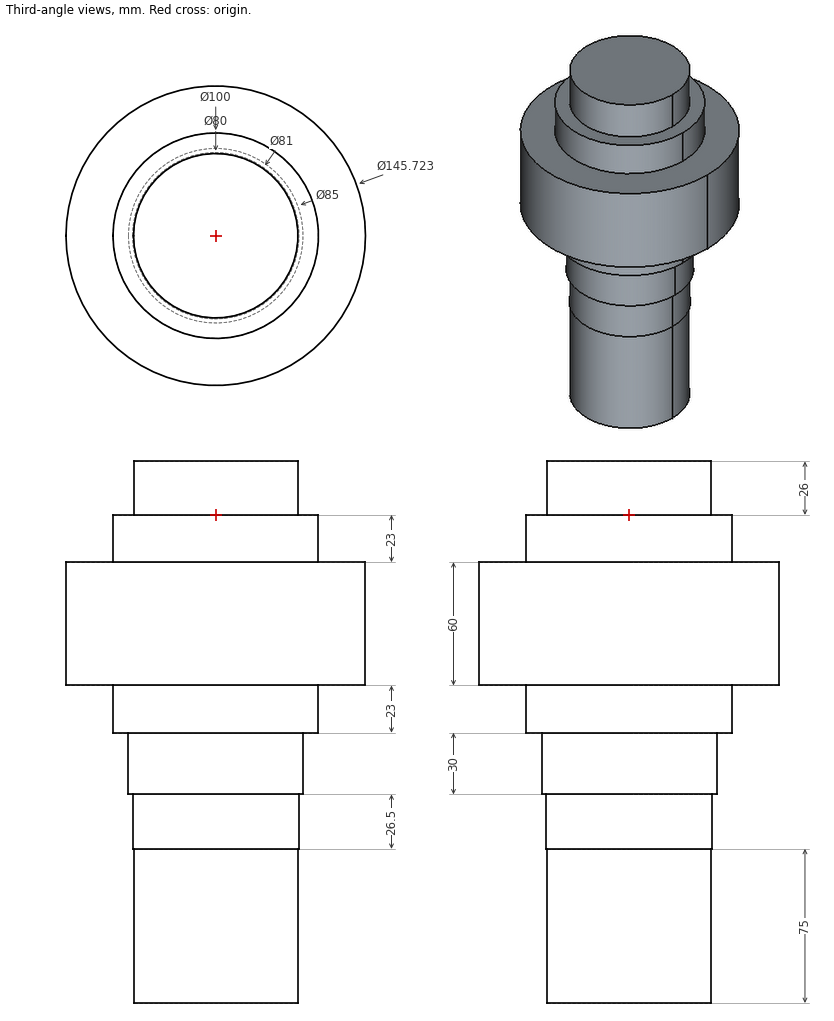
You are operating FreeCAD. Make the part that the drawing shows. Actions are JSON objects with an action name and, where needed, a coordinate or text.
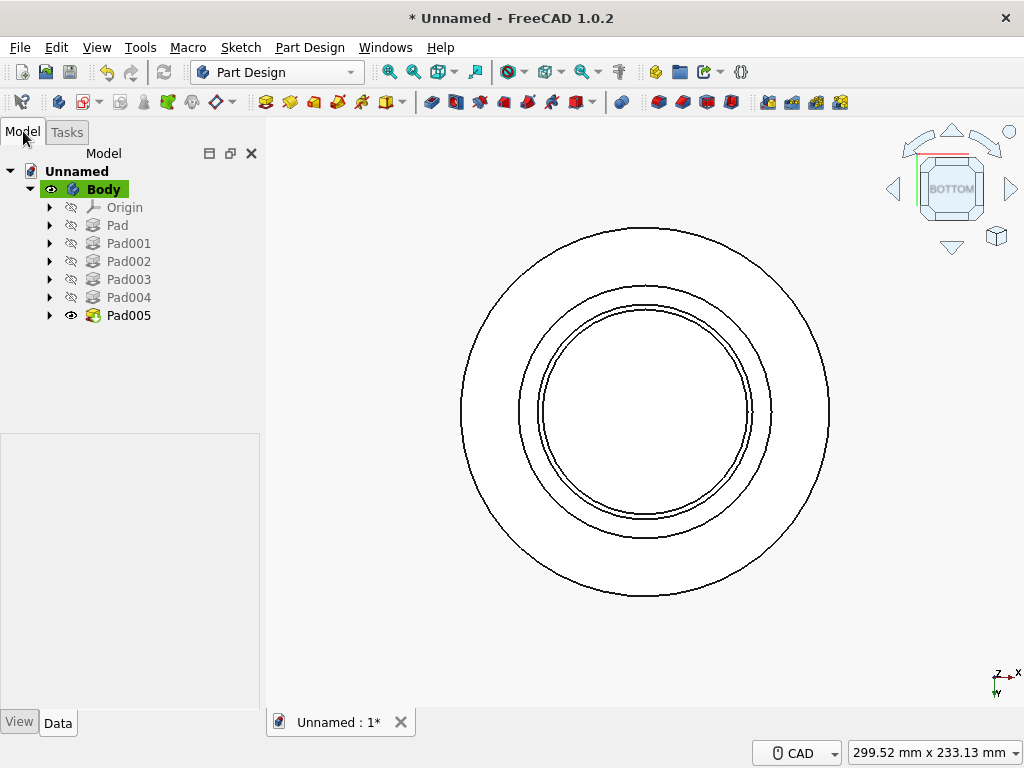
{"action": "left_click", "coordinate": [50, 207]}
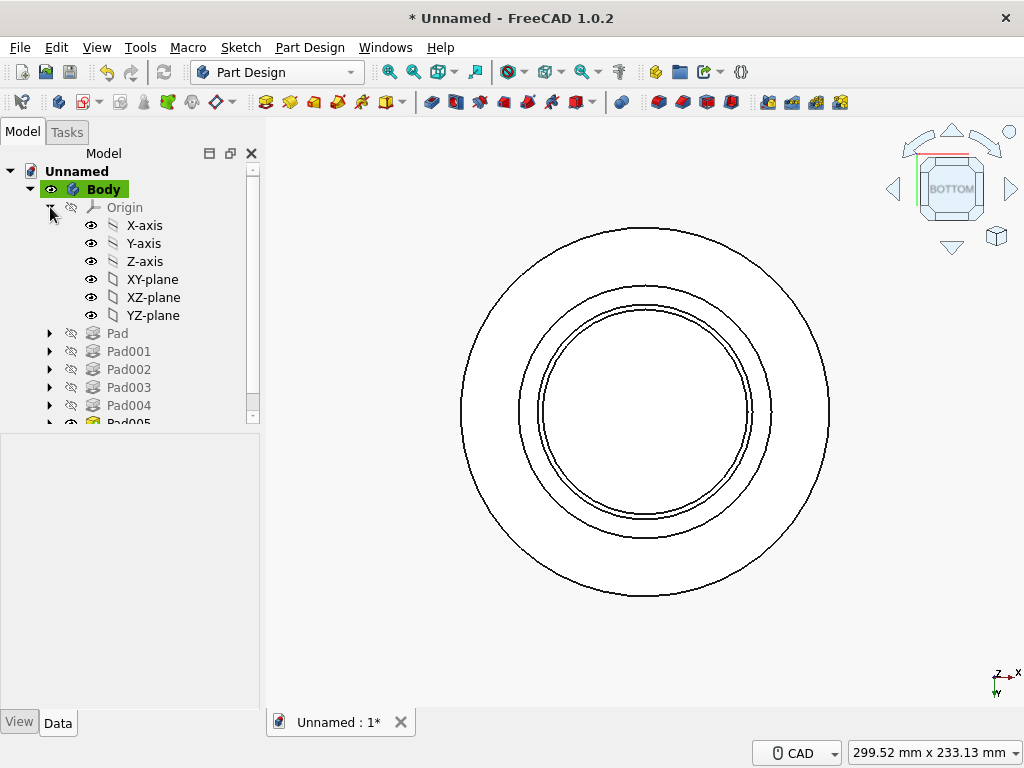
{"action": "left_click", "coordinate": [136, 279]}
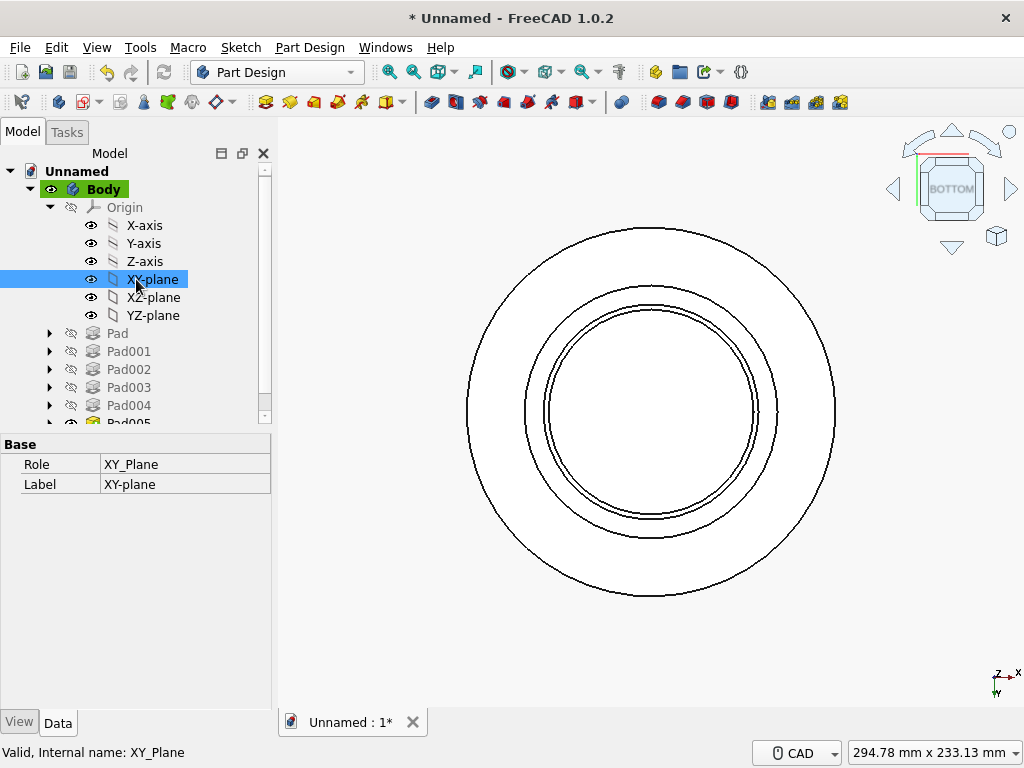
{"action": "left_click", "coordinate": [216, 102]}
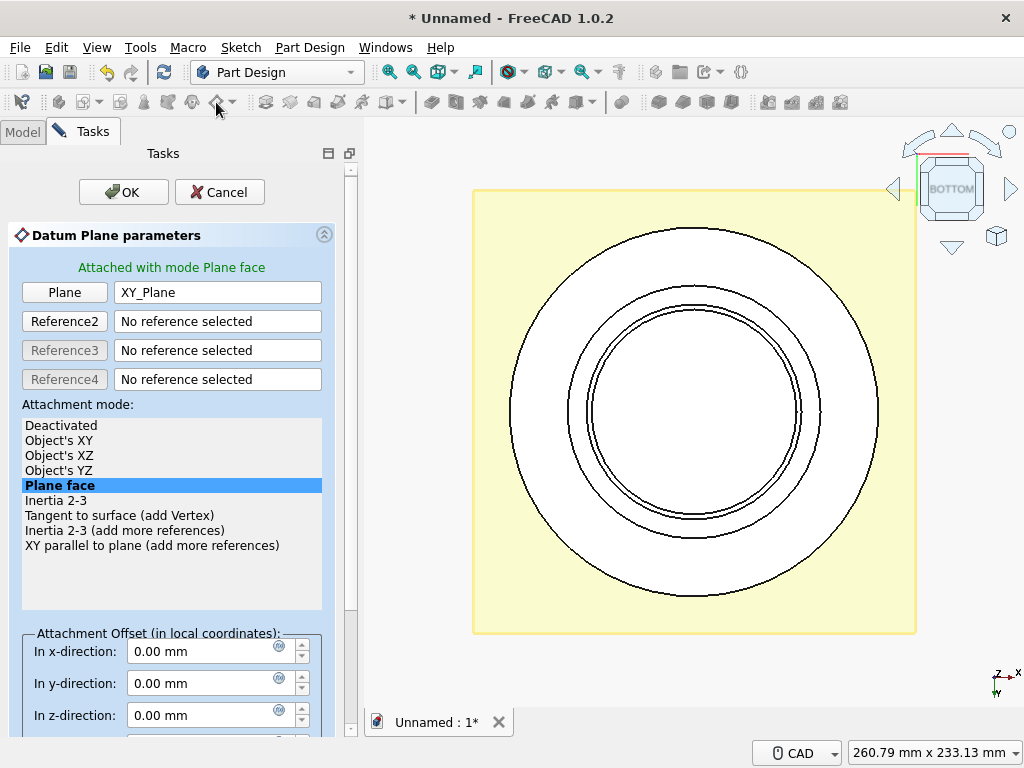
{"action": "triple_click", "coordinate": [210, 715]}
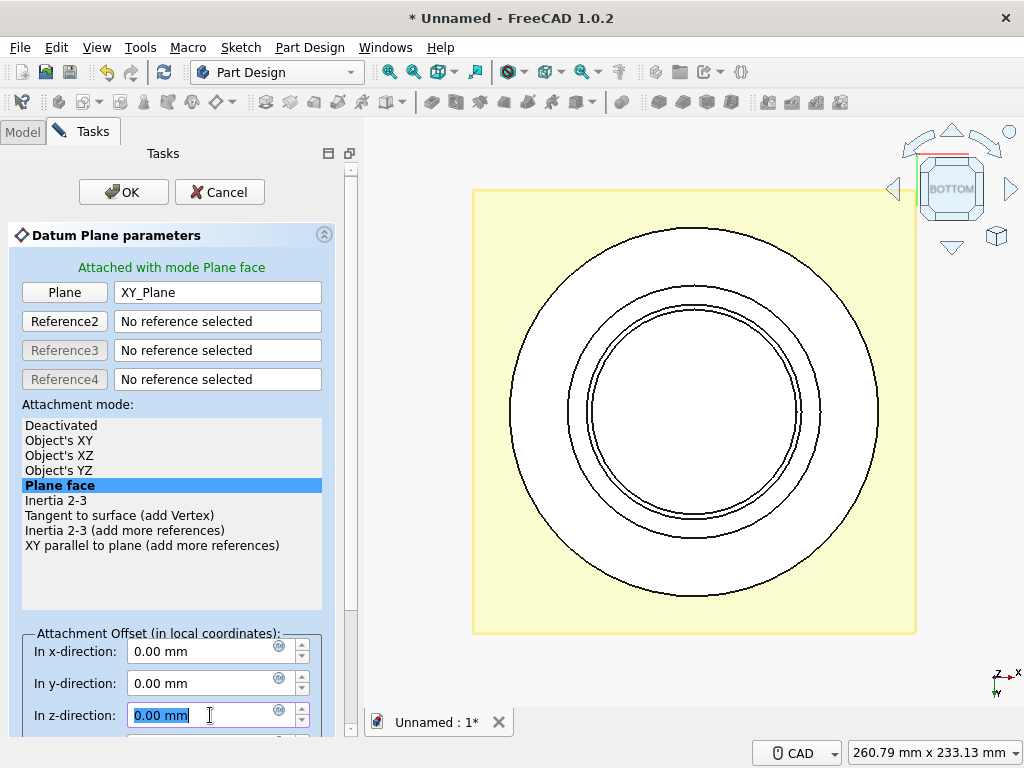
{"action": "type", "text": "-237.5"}
{"action": "key", "text": "Tab"}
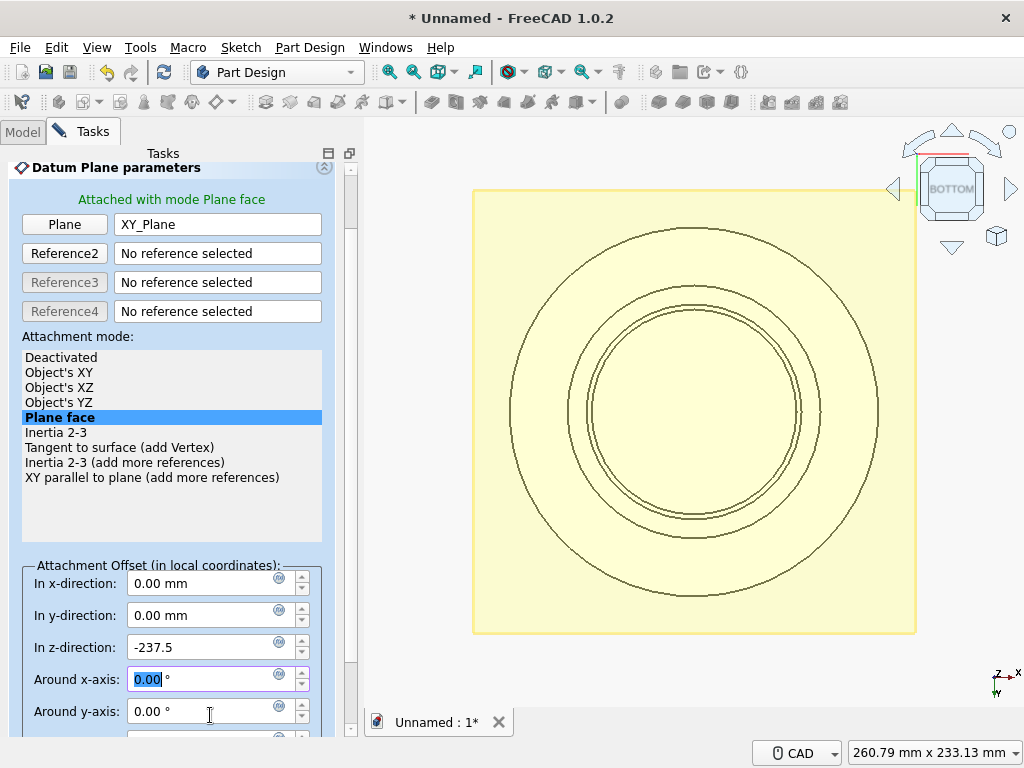
{"action": "scroll", "coordinate": [351, 450], "scroll_direction": "up", "scroll_amount": 2}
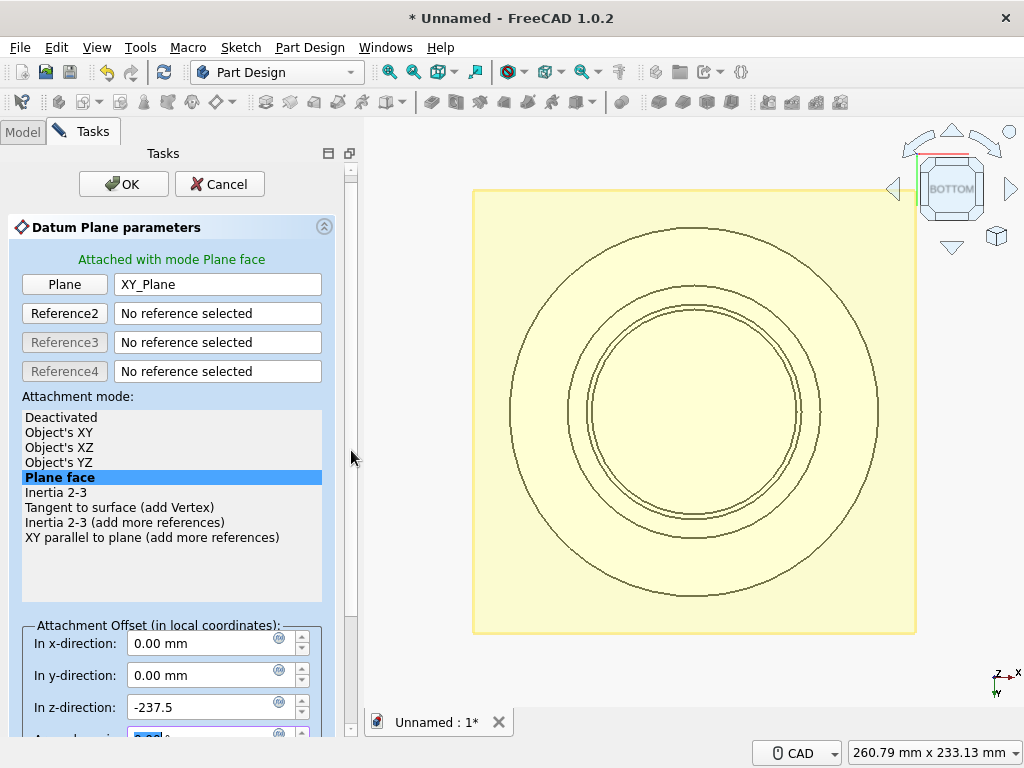
{"action": "left_click", "coordinate": [124, 192]}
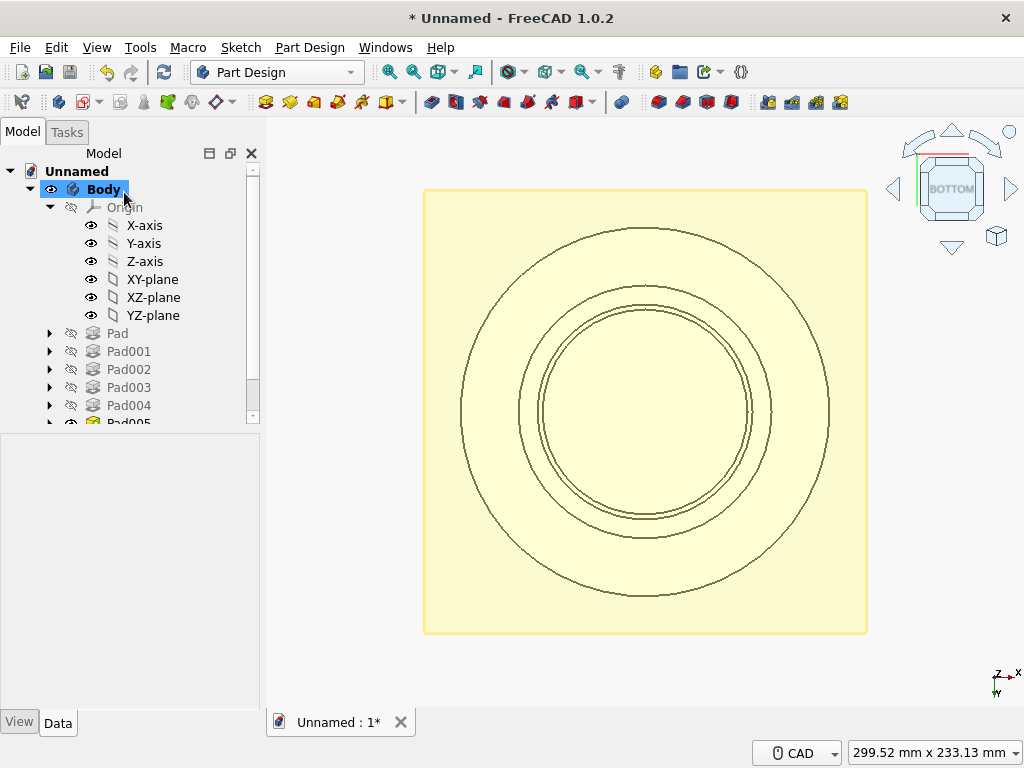
{"action": "scroll", "coordinate": [100, 293], "scroll_direction": "down", "scroll_amount": 3}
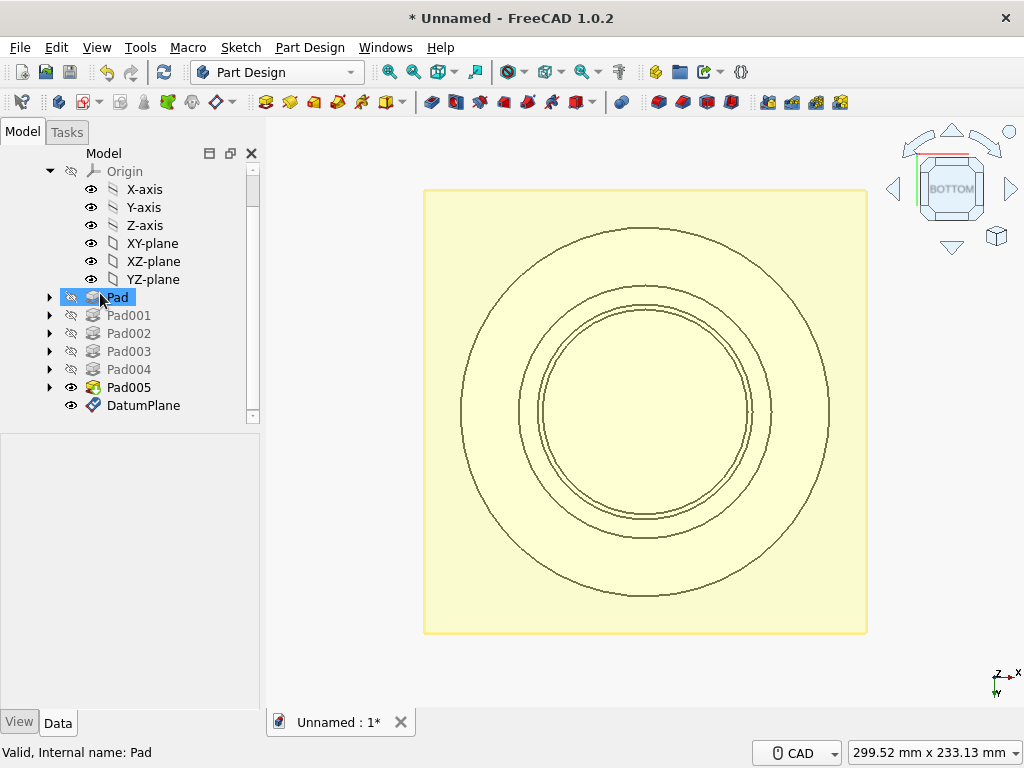
{"action": "left_click", "coordinate": [116, 405]}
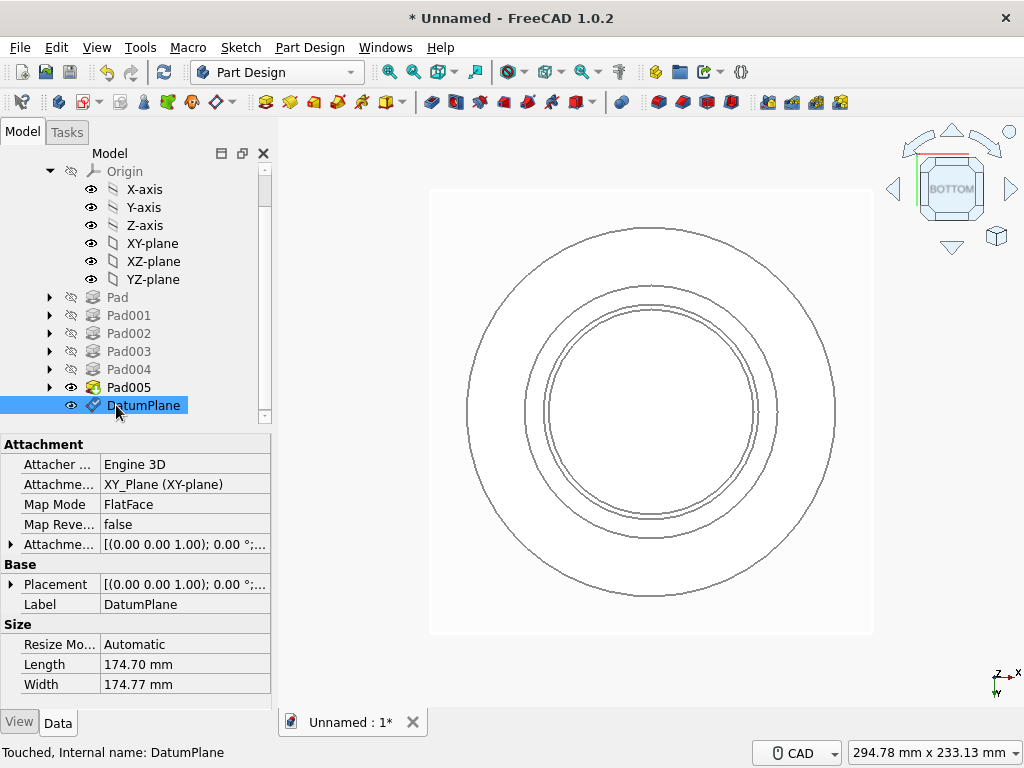
{"action": "left_click", "coordinate": [84, 102]}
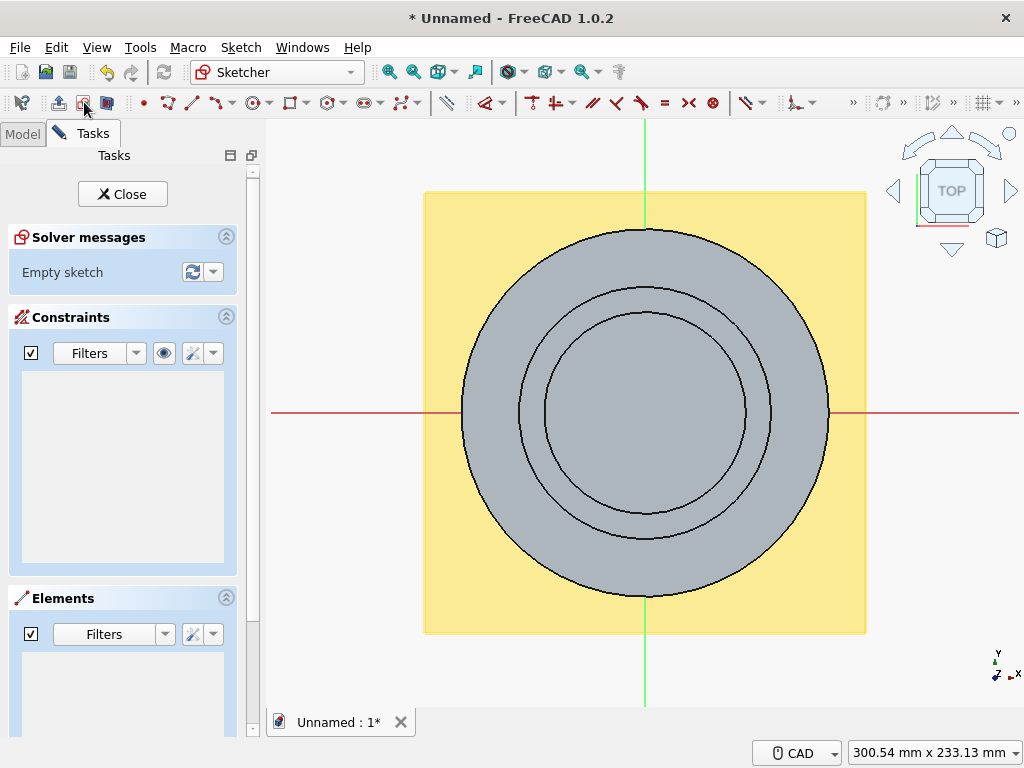
{"action": "key", "text": "q s"}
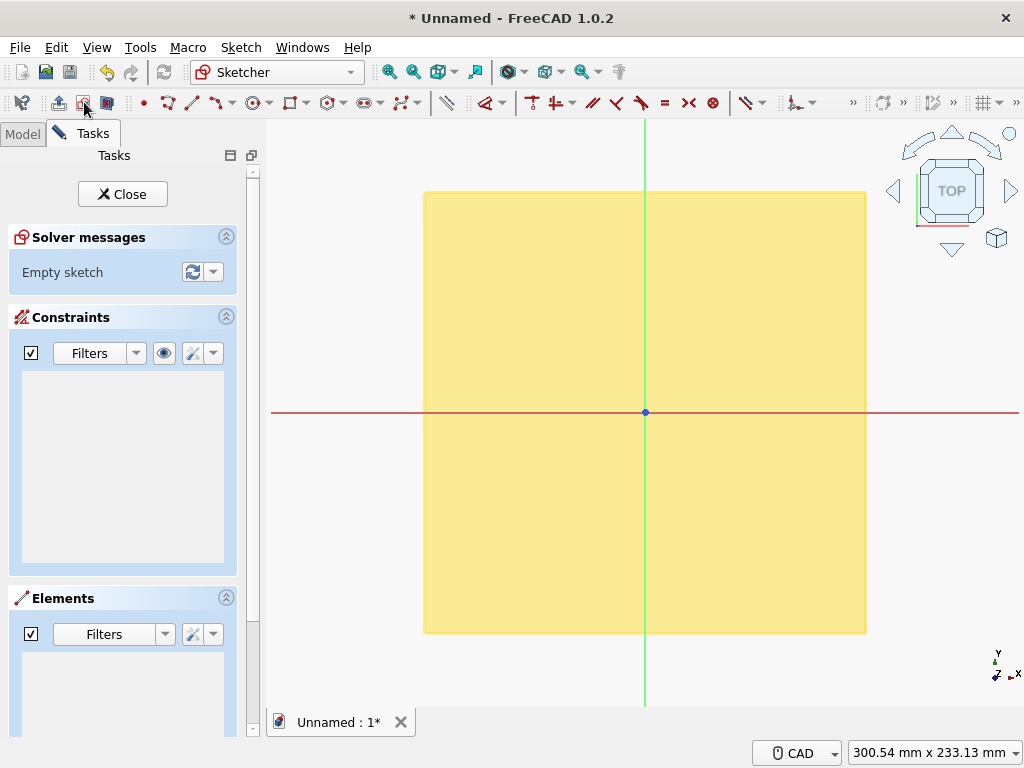
{"action": "scroll", "coordinate": [728, 413], "scroll_direction": "up", "scroll_amount": 3}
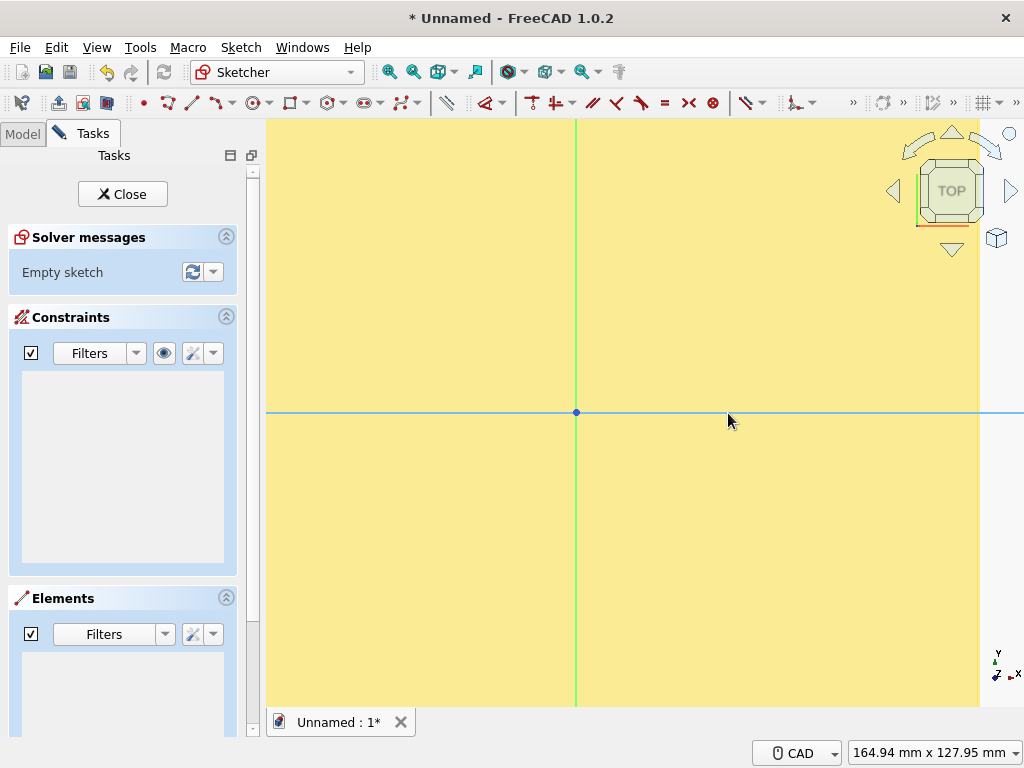
{"action": "key", "text": "g c"}